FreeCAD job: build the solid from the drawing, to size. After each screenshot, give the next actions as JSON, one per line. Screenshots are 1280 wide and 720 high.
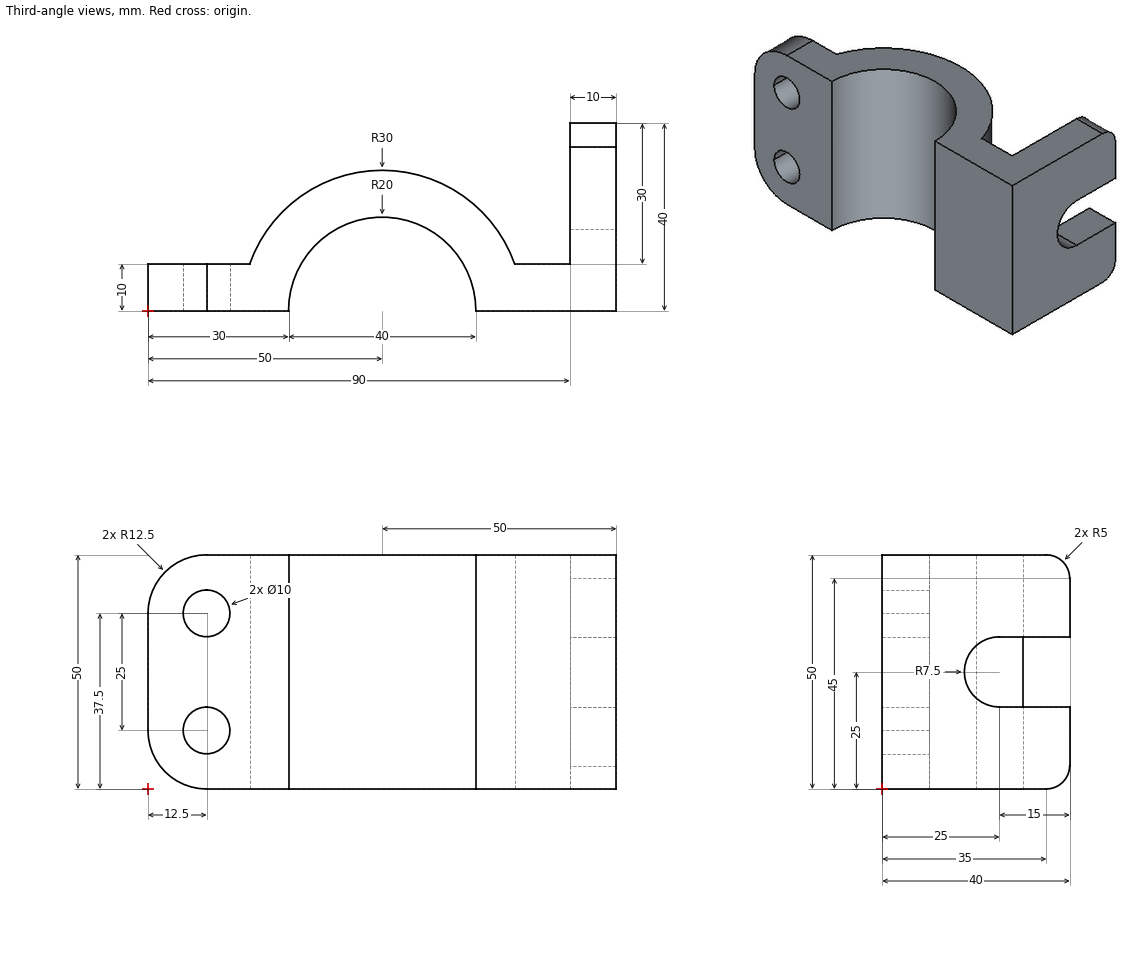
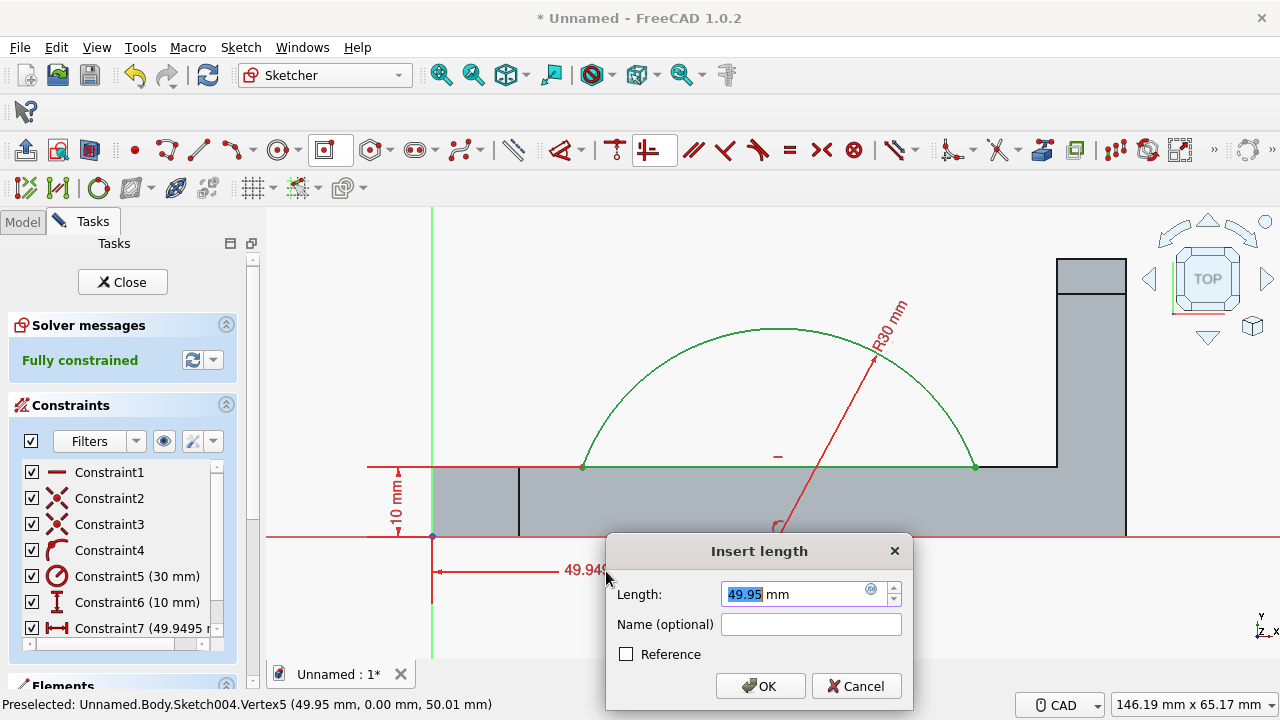
{"action": "type", "text": "50"}
{"action": "key", "text": "Return"}
{"action": "key", "text": "Escape"}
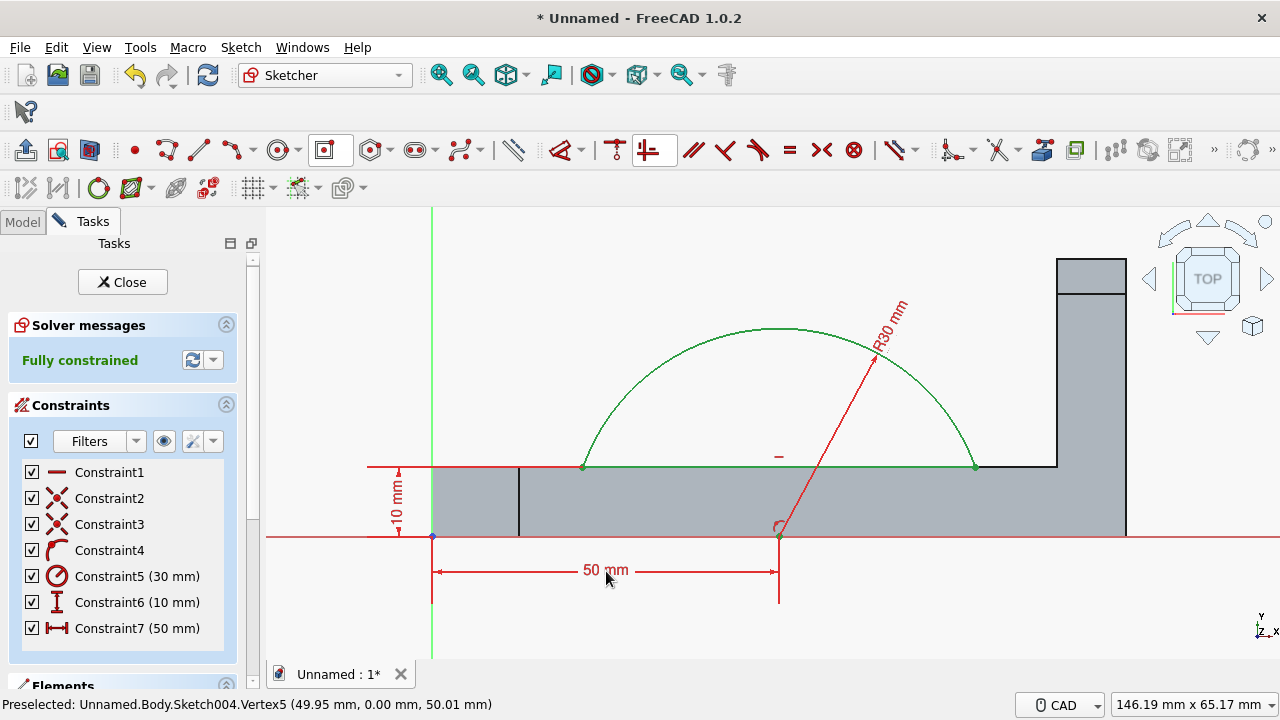
{"action": "left_click", "coordinate": [123, 282]}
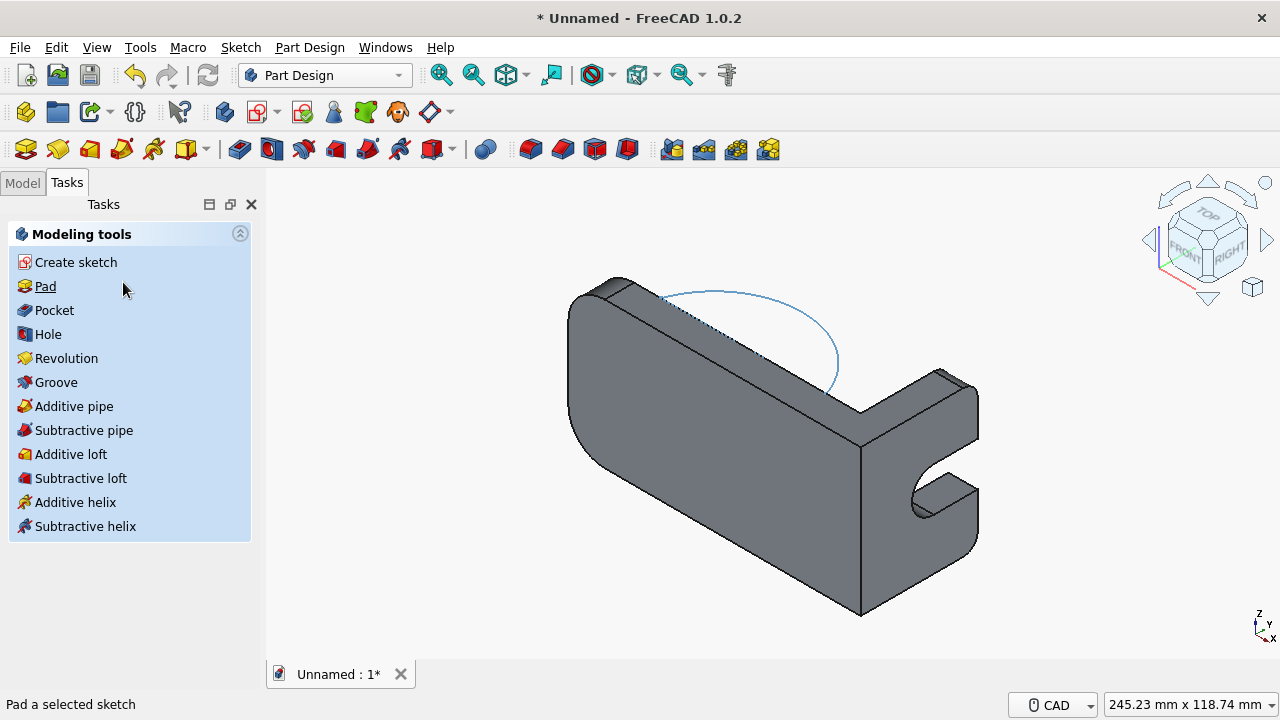
{"action": "left_click", "coordinate": [26, 150]}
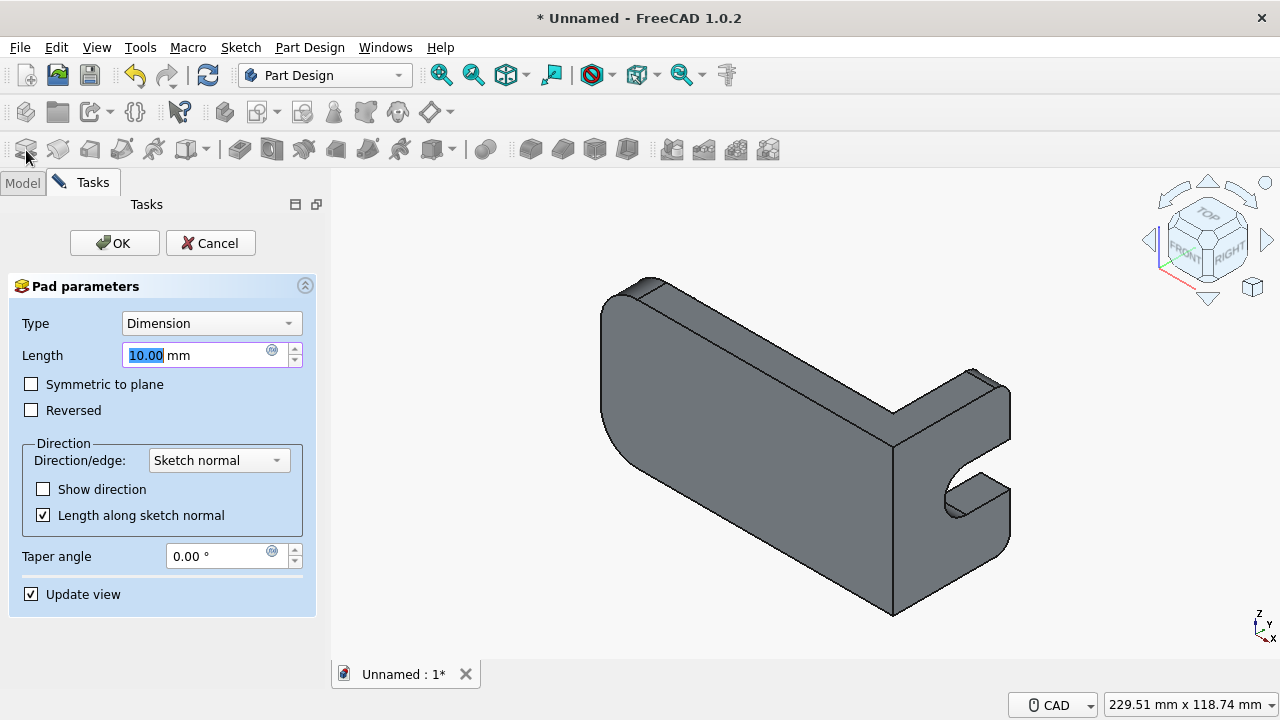
{"action": "type", "text": "50"}
{"action": "key", "text": "Tab"}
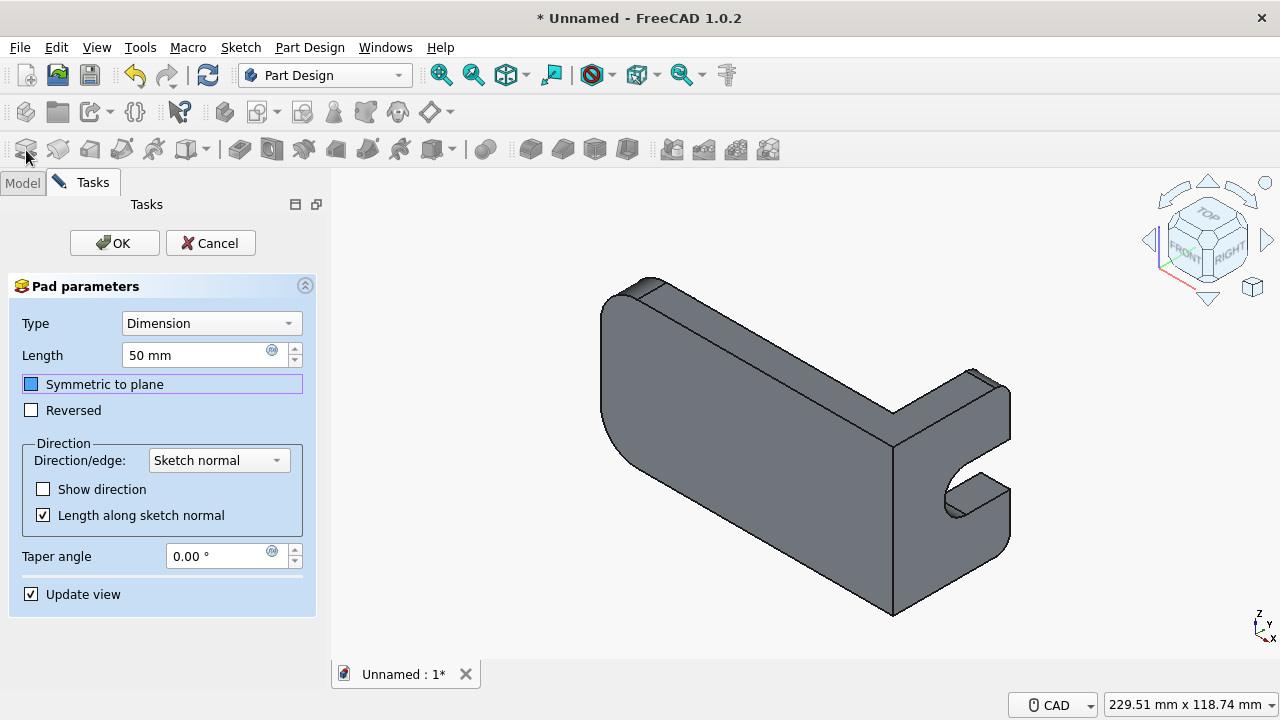
{"action": "left_click", "coordinate": [30, 410]}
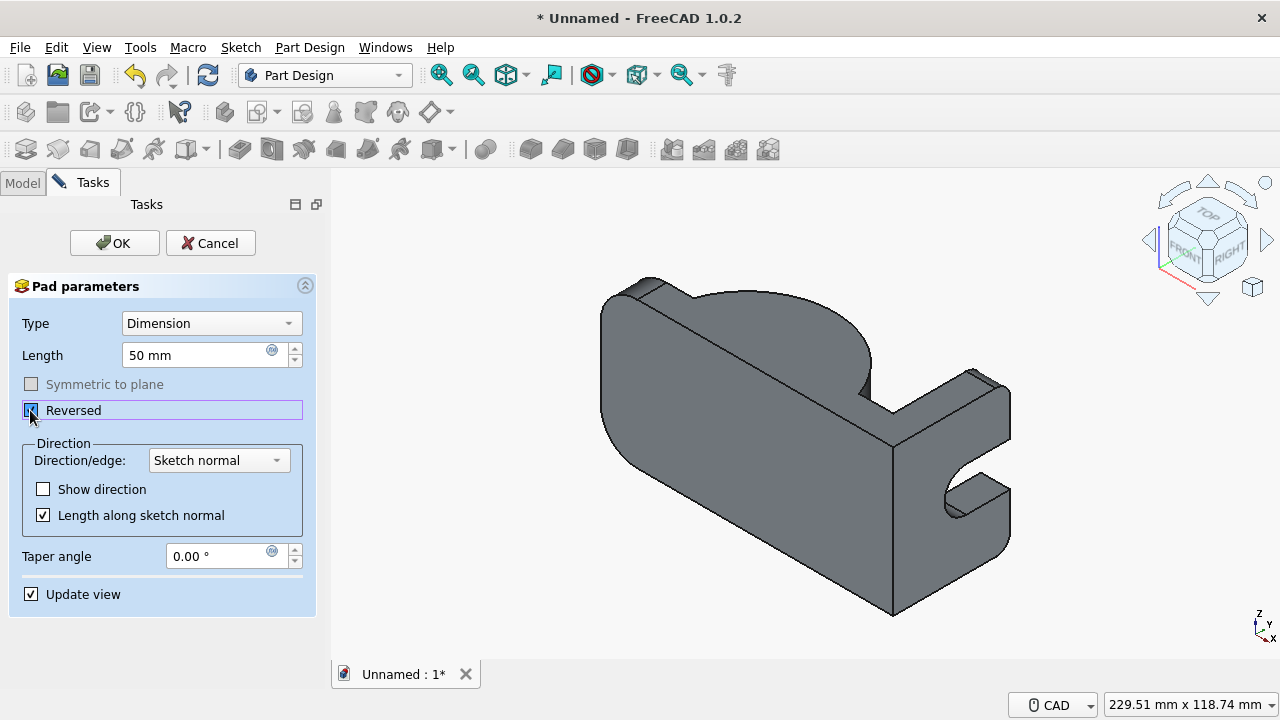
{"action": "left_click", "coordinate": [115, 243]}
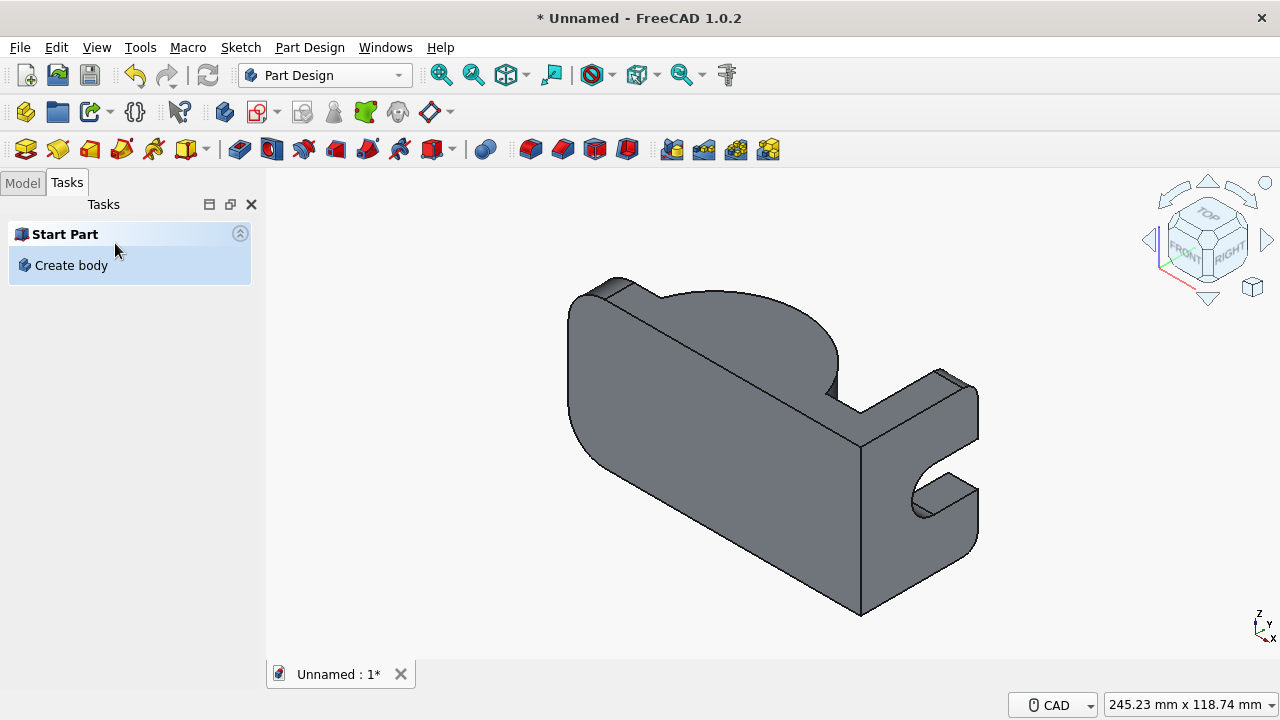
{"action": "left_click", "coordinate": [769, 351]}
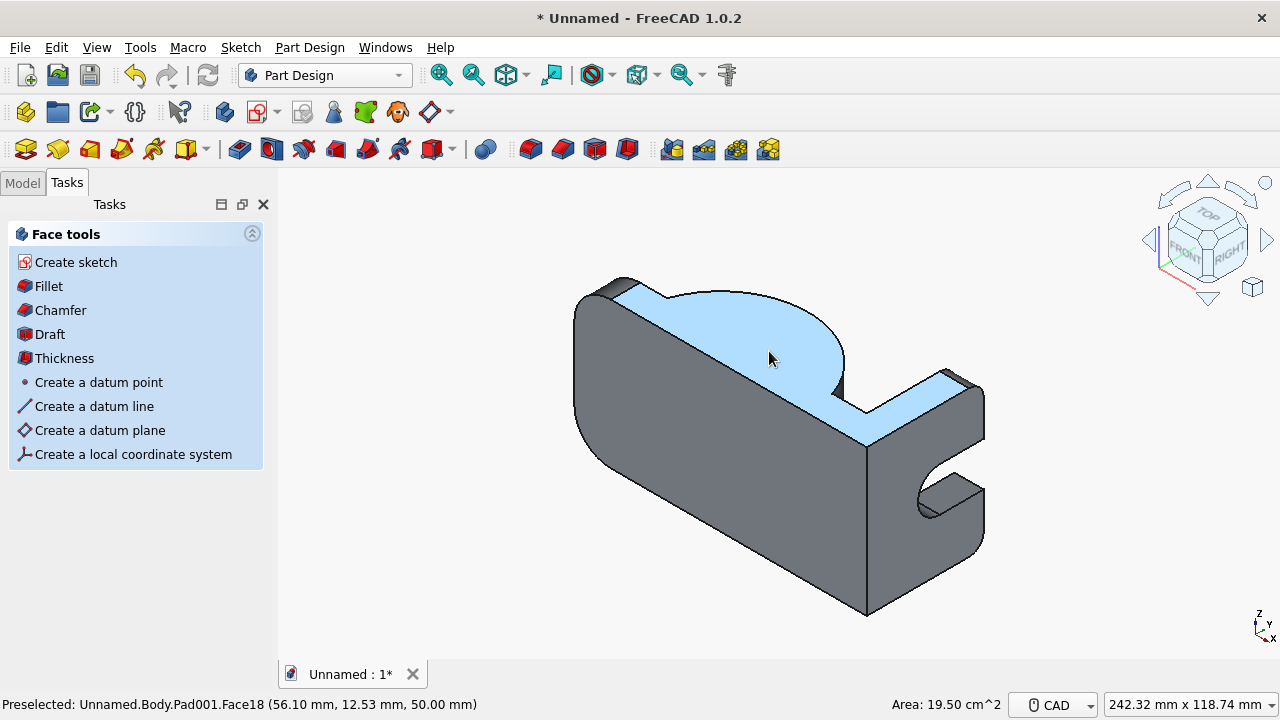
{"action": "left_click", "coordinate": [258, 112]}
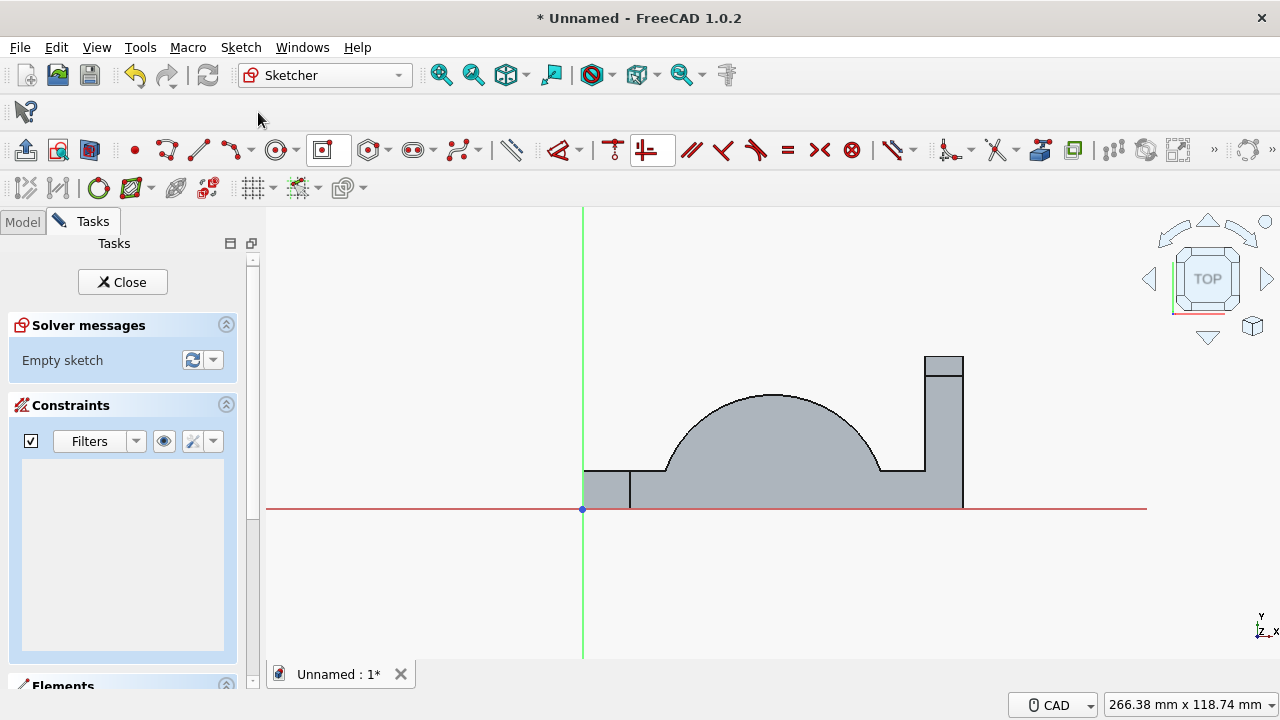
{"action": "scroll", "coordinate": [725, 502], "scroll_direction": "up", "scroll_amount": 4}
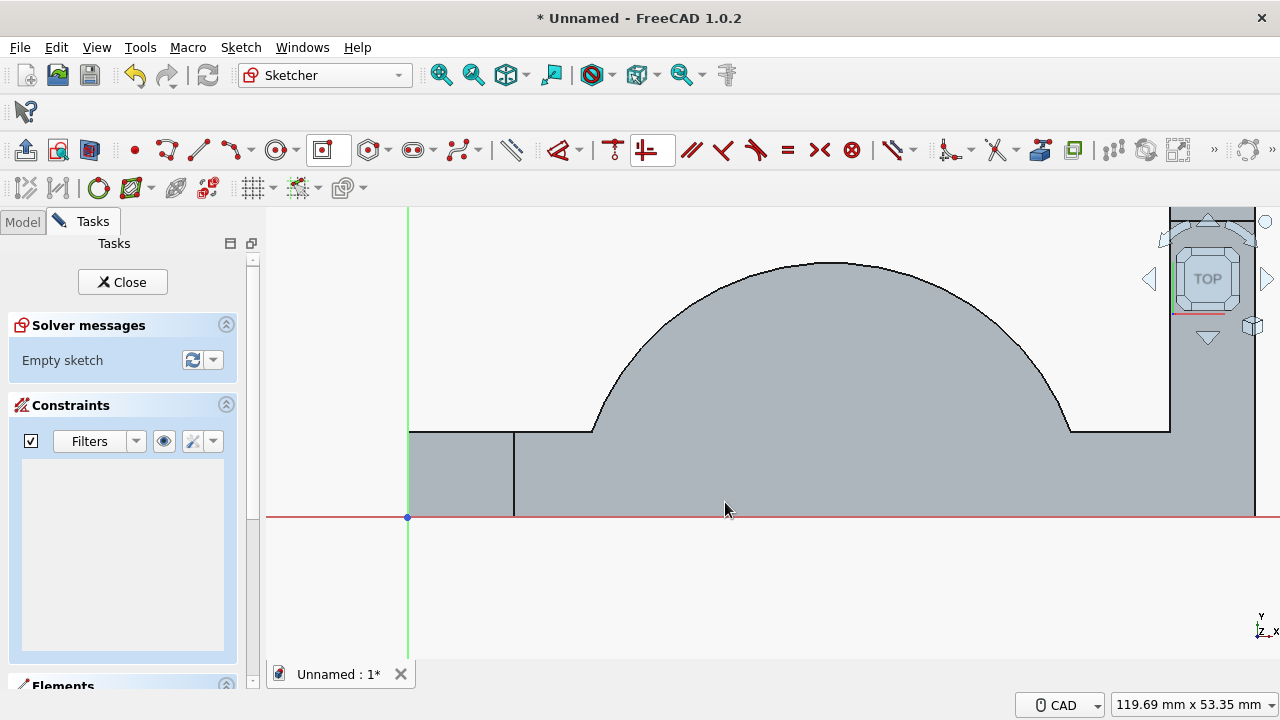
{"action": "left_click", "coordinate": [200, 150]}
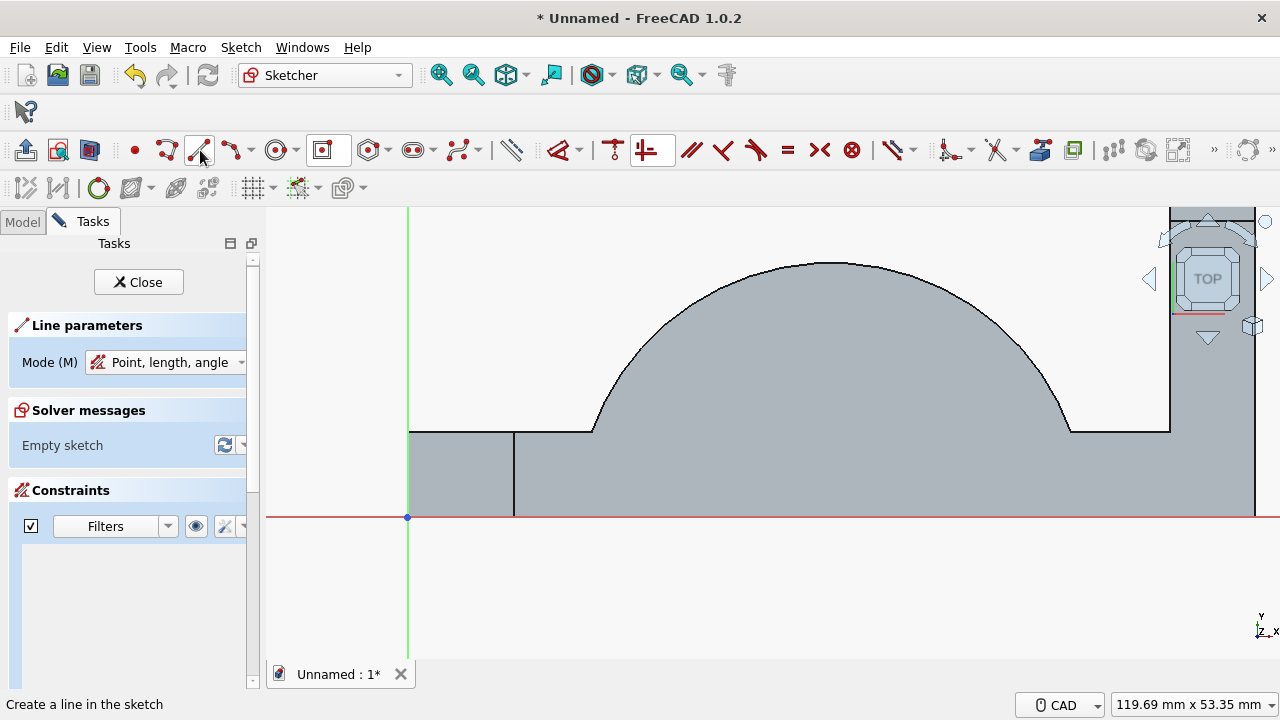
{"action": "left_click", "coordinate": [662, 517]}
{"action": "left_click", "coordinate": [1001, 508]}